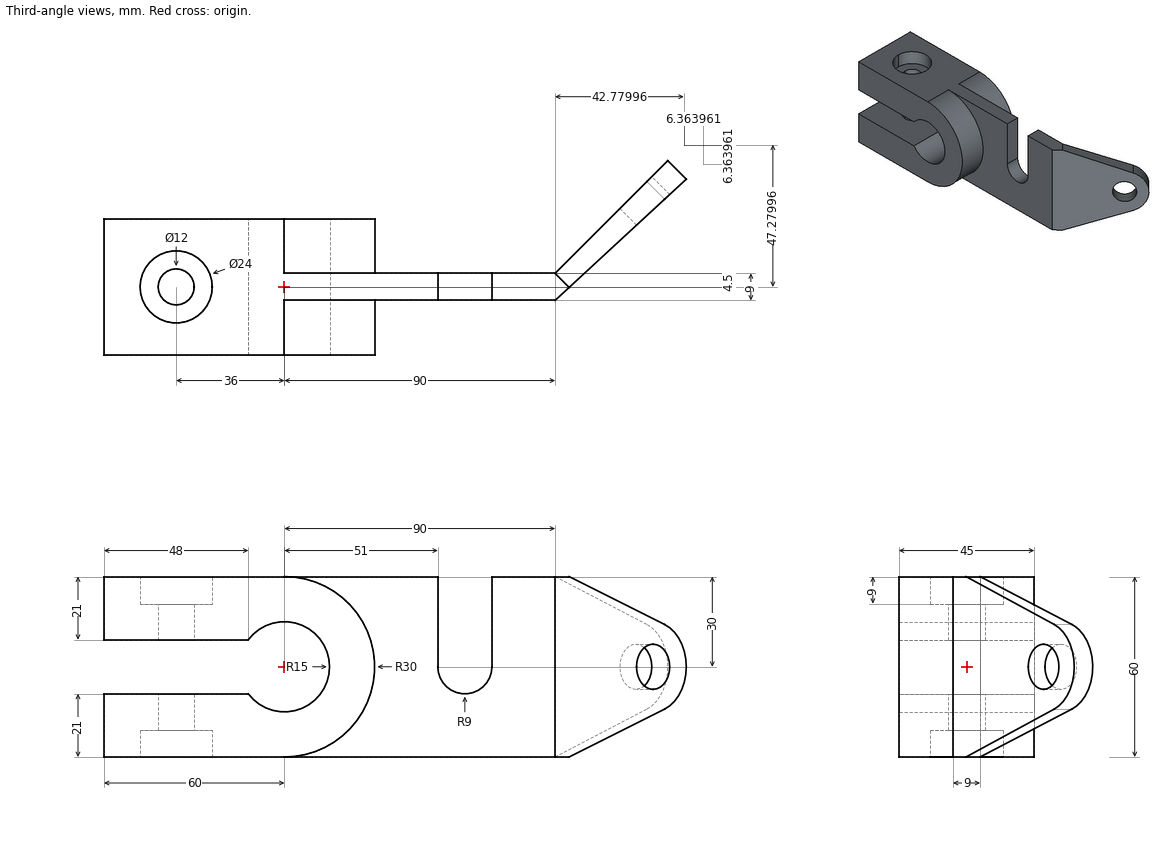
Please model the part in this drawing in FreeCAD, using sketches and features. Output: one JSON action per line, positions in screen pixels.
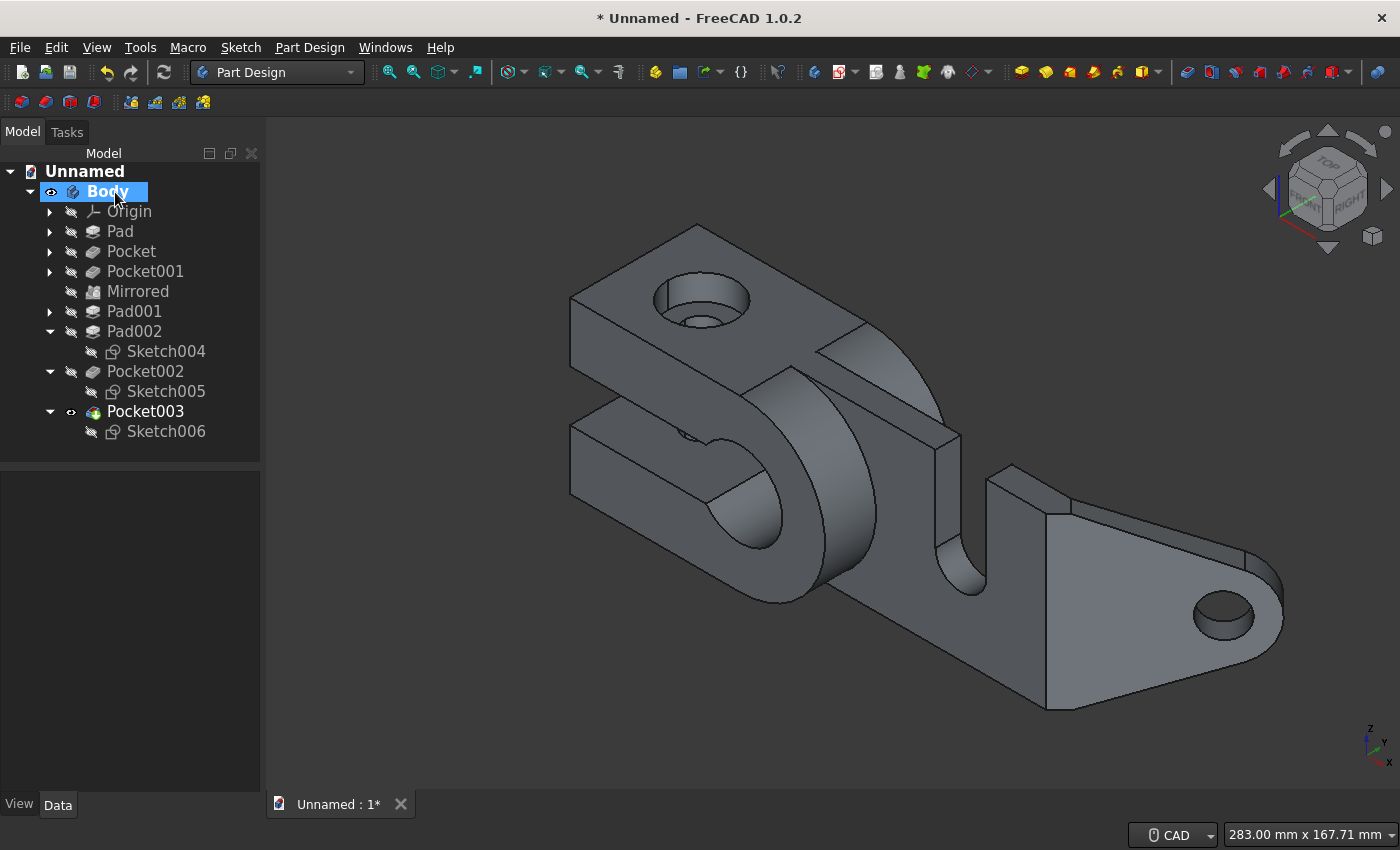
{"action": "key", "text": "v f"}